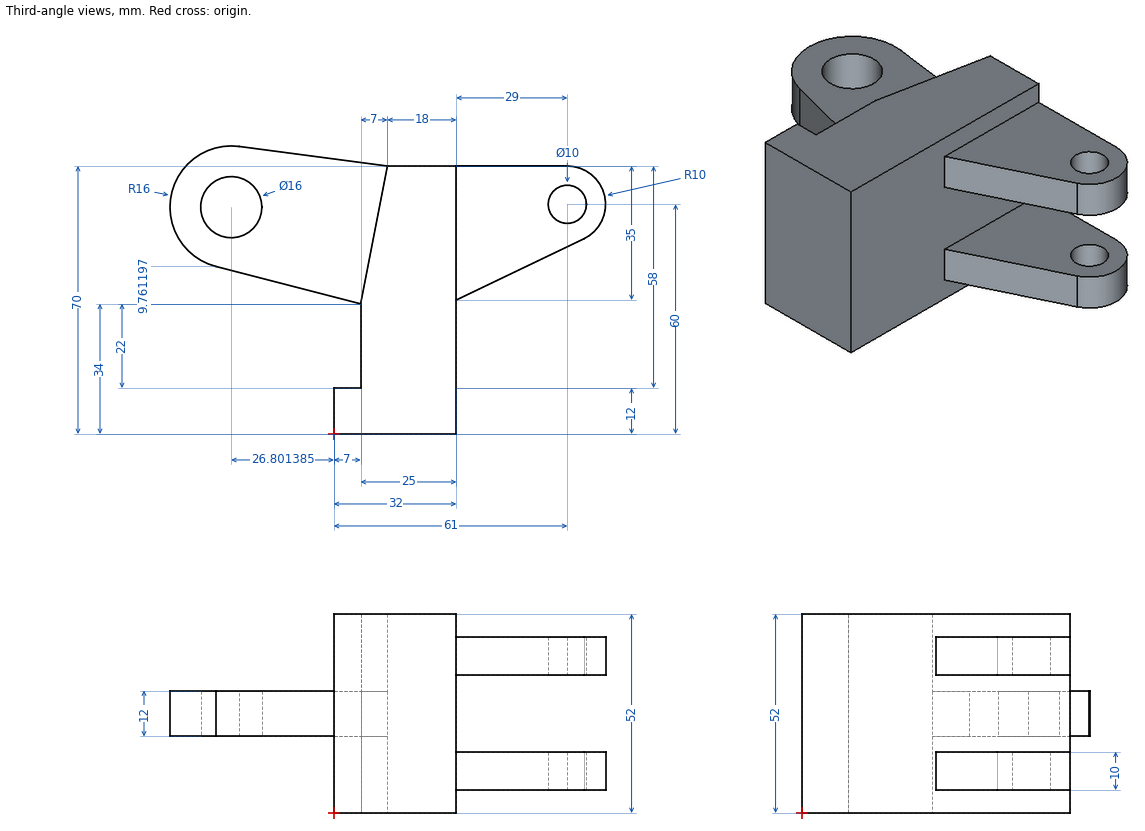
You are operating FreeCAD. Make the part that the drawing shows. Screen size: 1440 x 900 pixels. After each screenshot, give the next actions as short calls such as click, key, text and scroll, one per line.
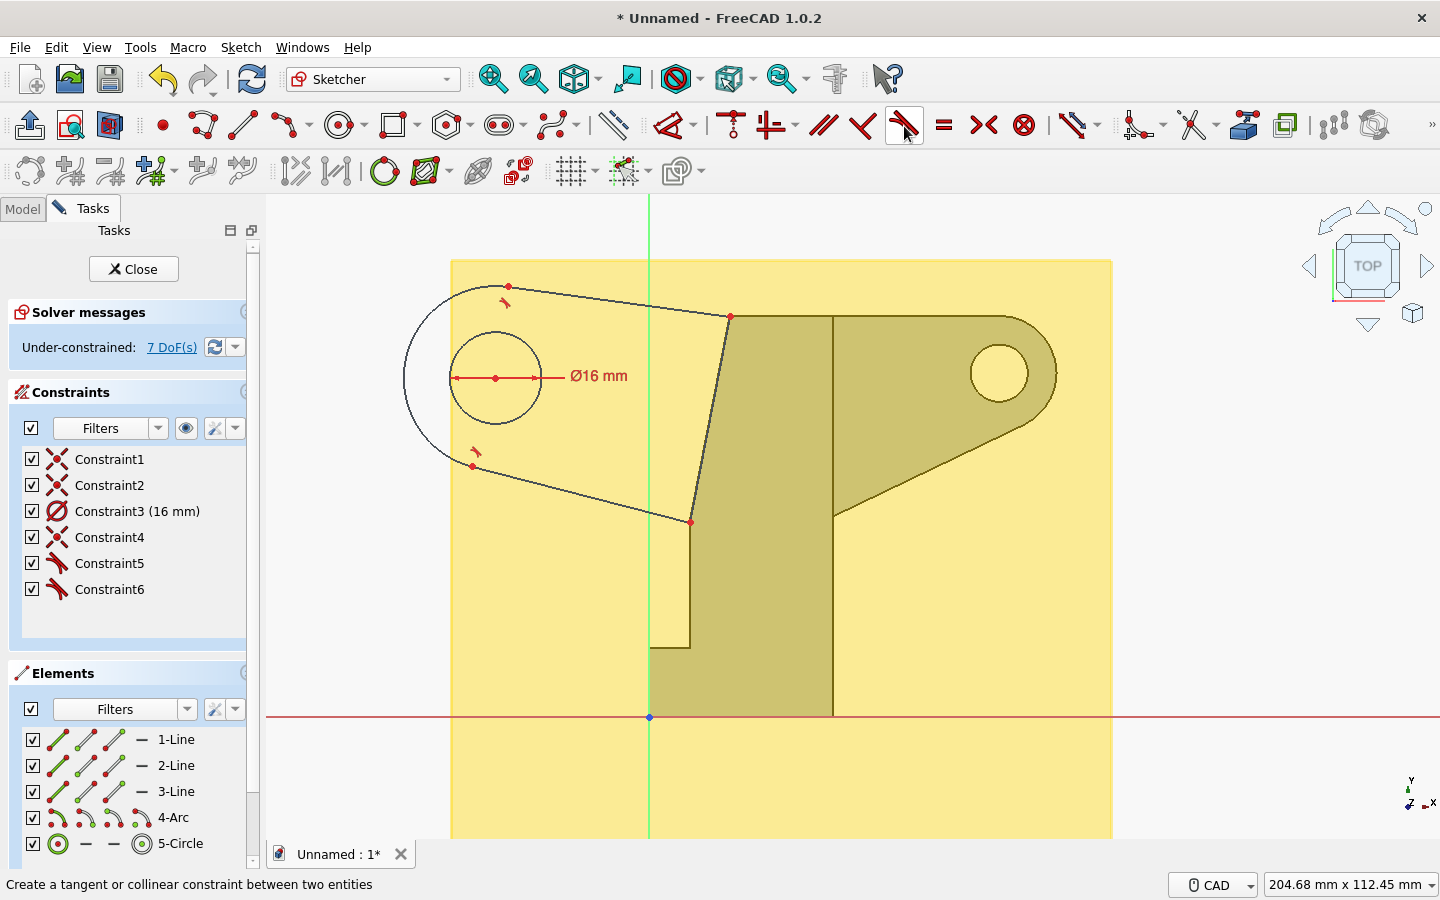
click(668, 126)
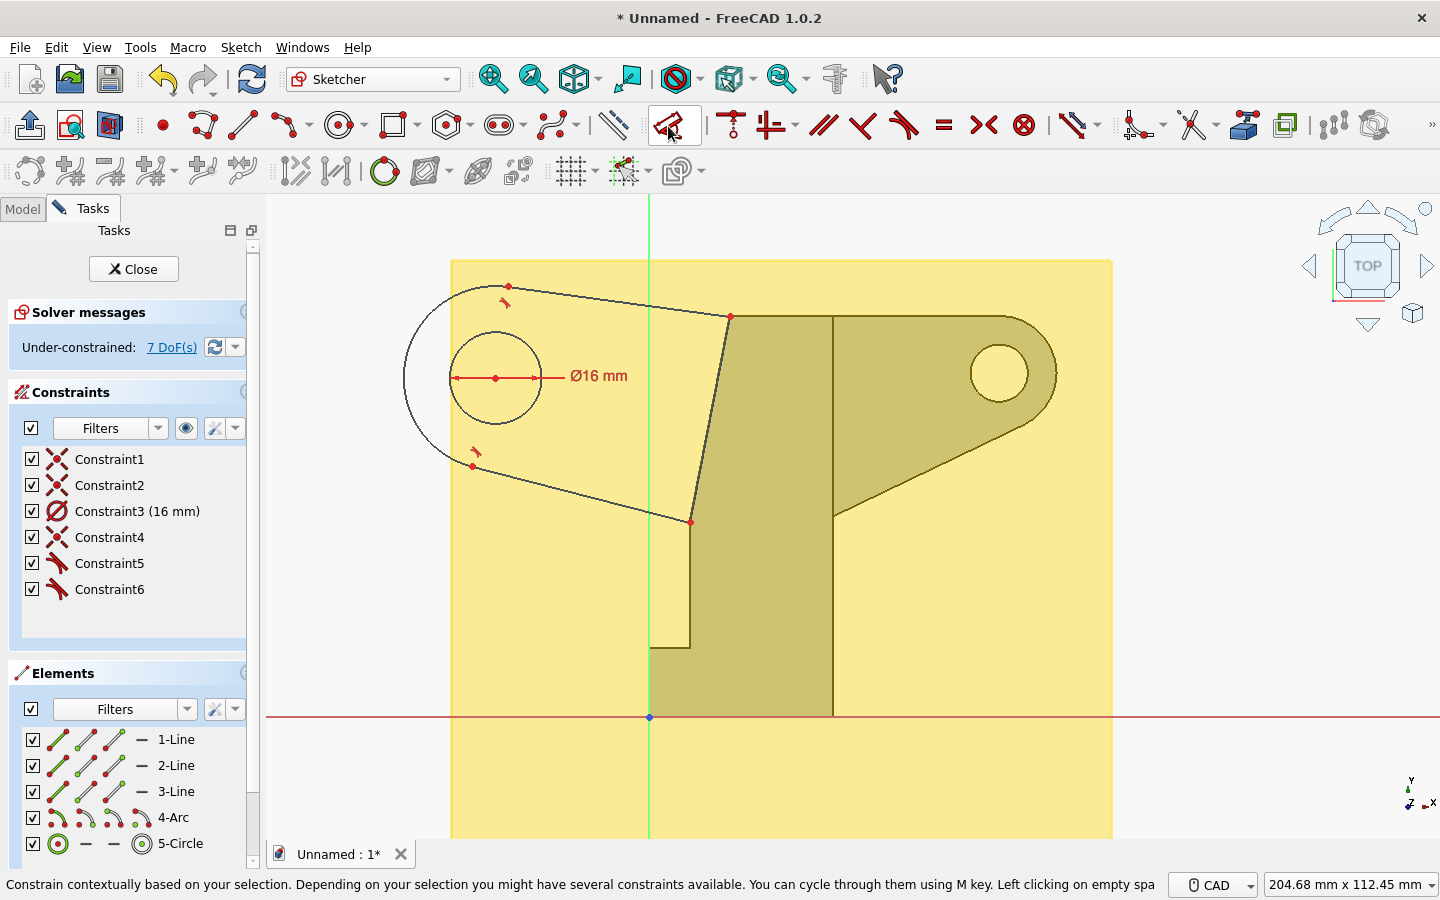
click(432, 312)
click(410, 289)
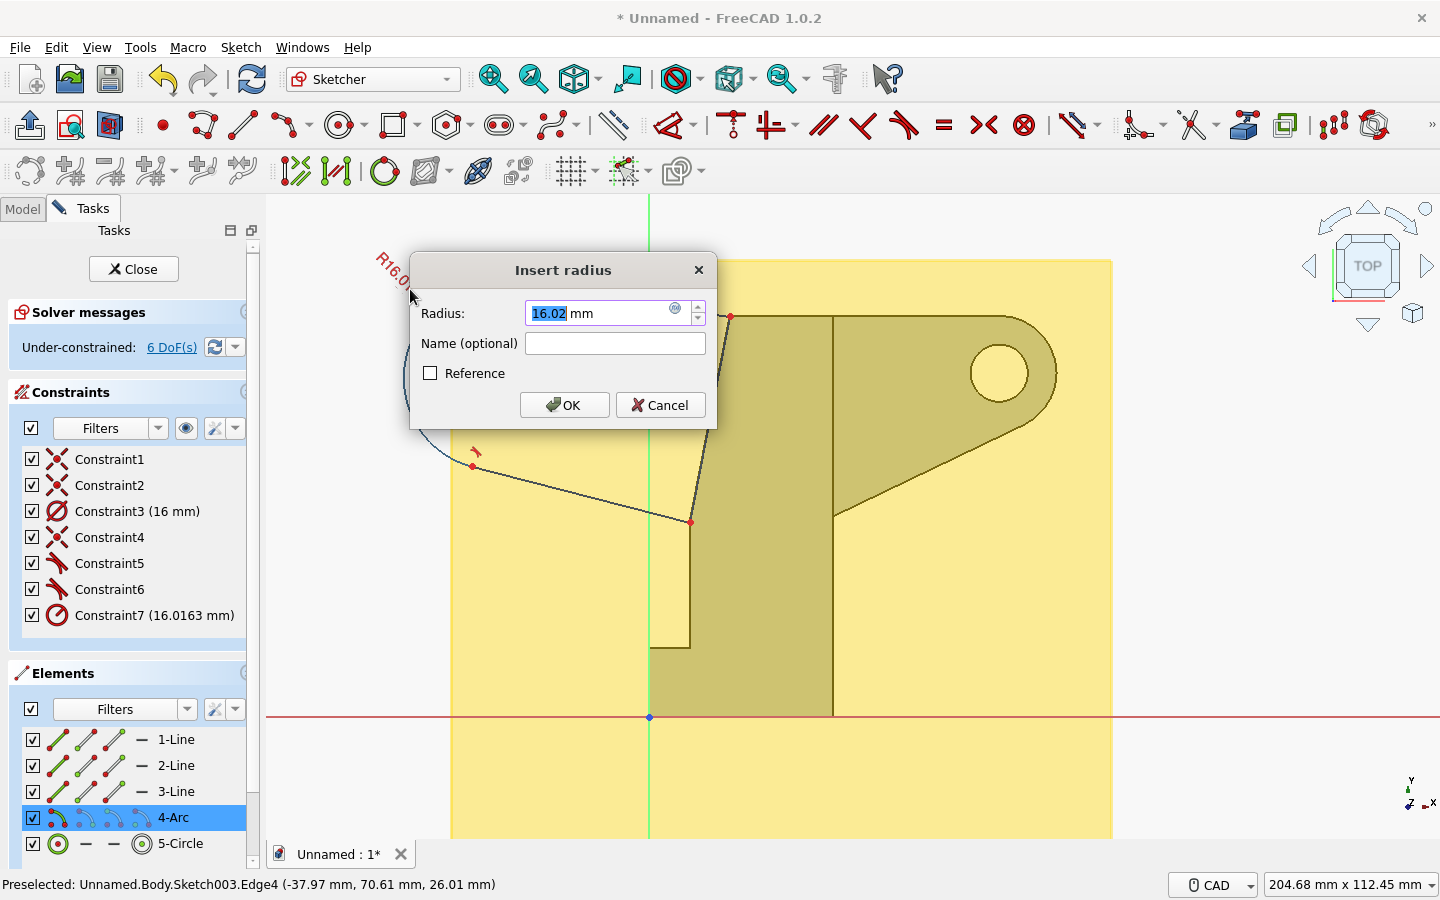
text(16)
key(Return)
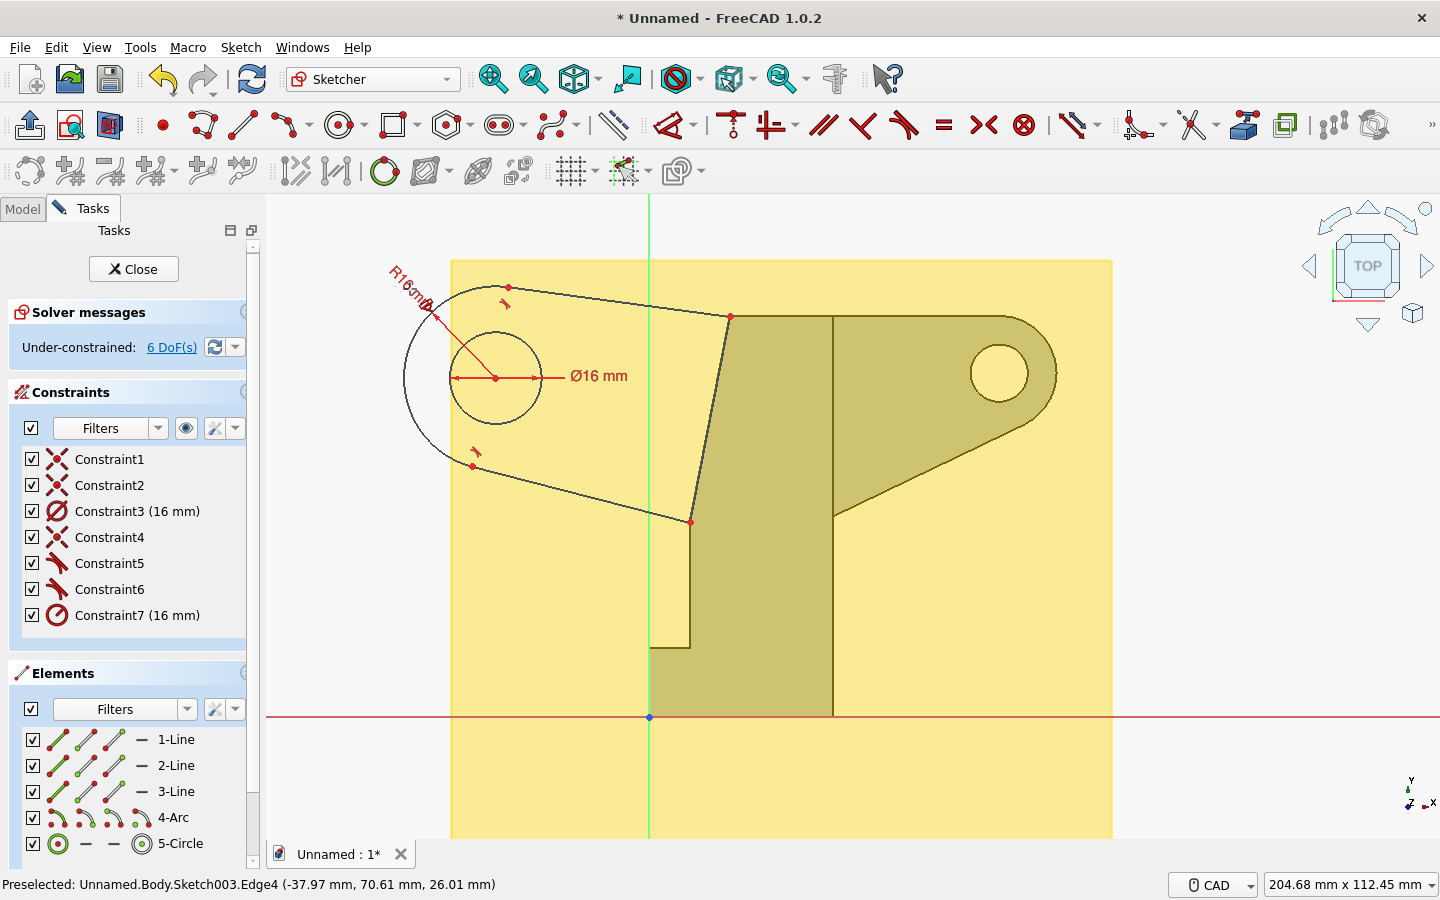
click(690, 523)
click(670, 751)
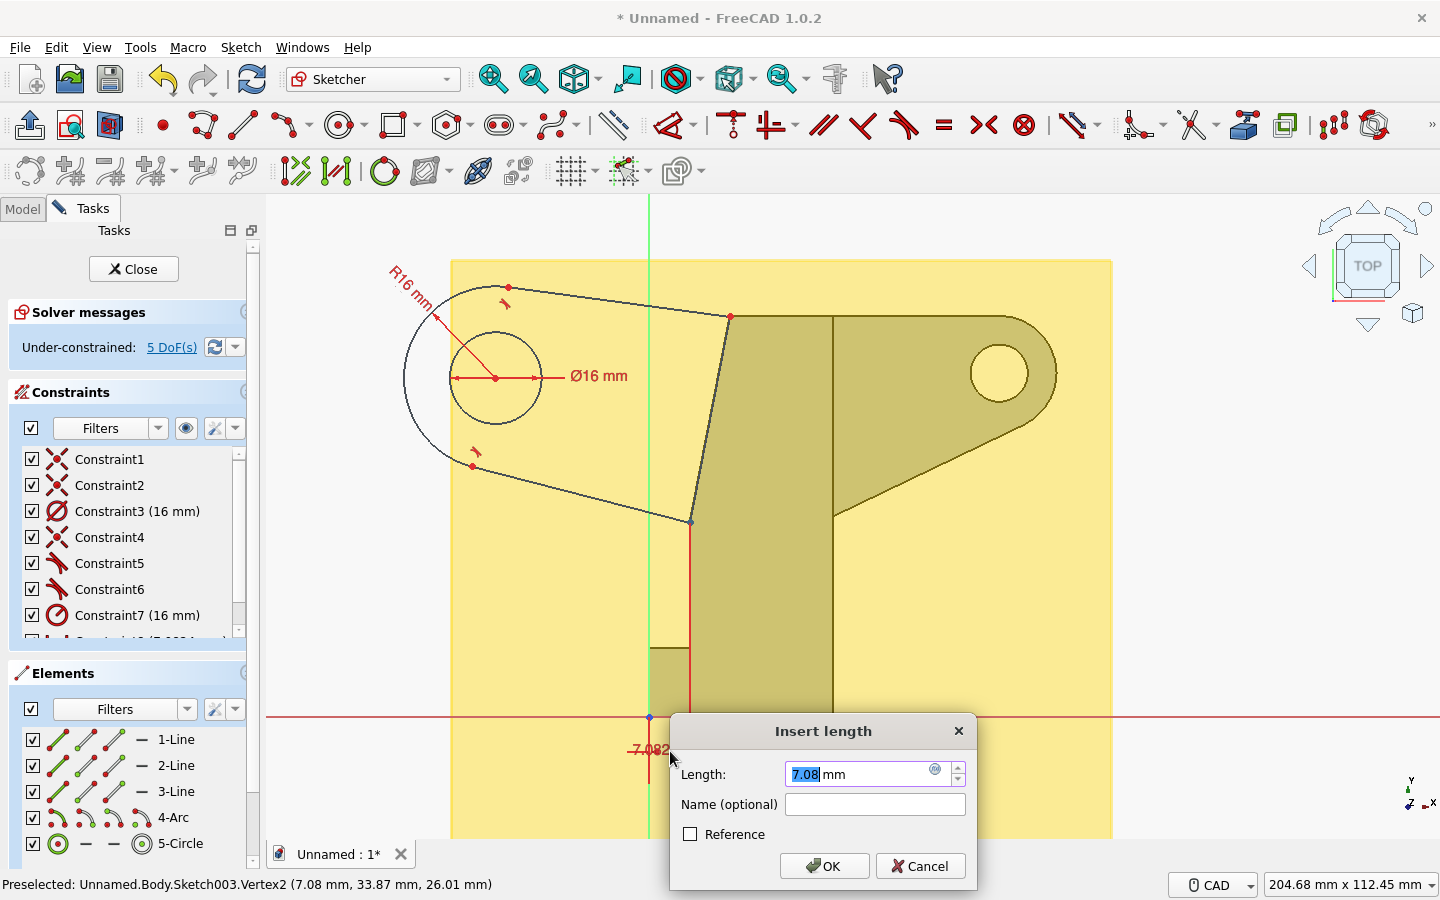
text(7)
key(Return)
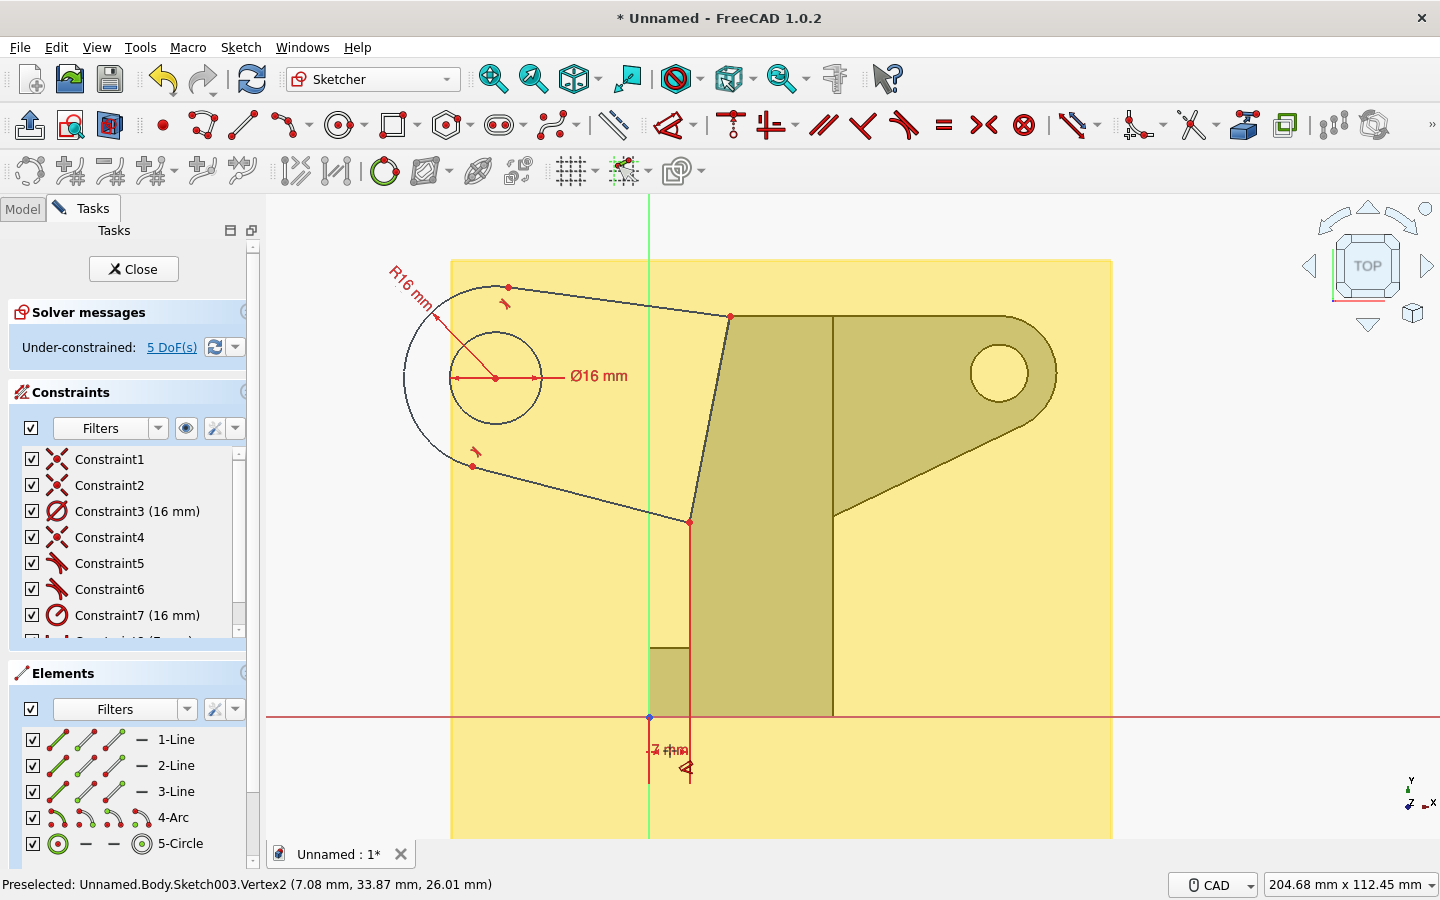
click(702, 461)
click(710, 283)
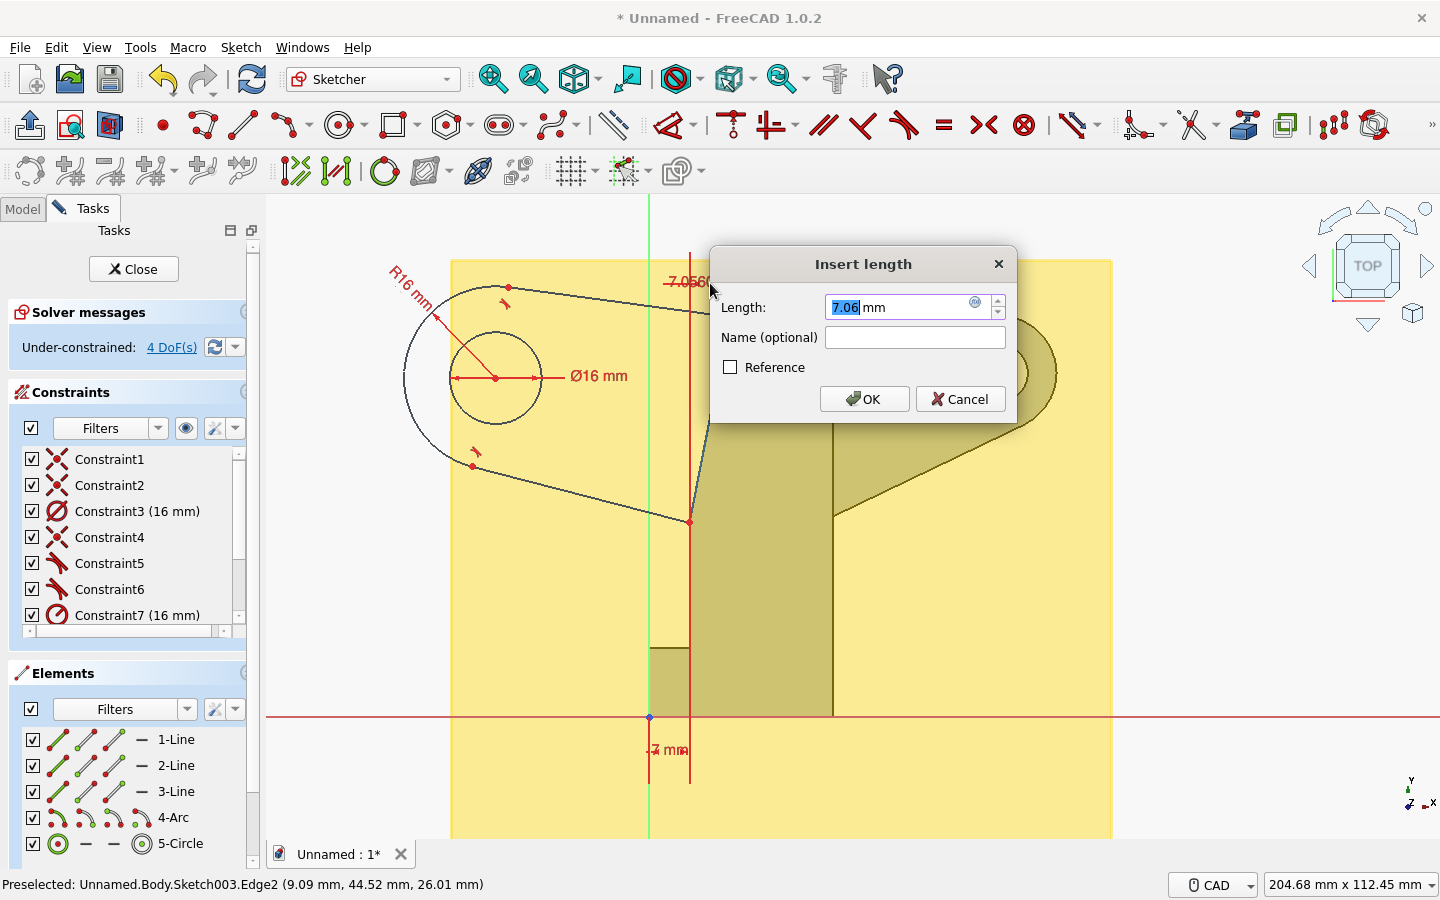
text(7)
key(Return)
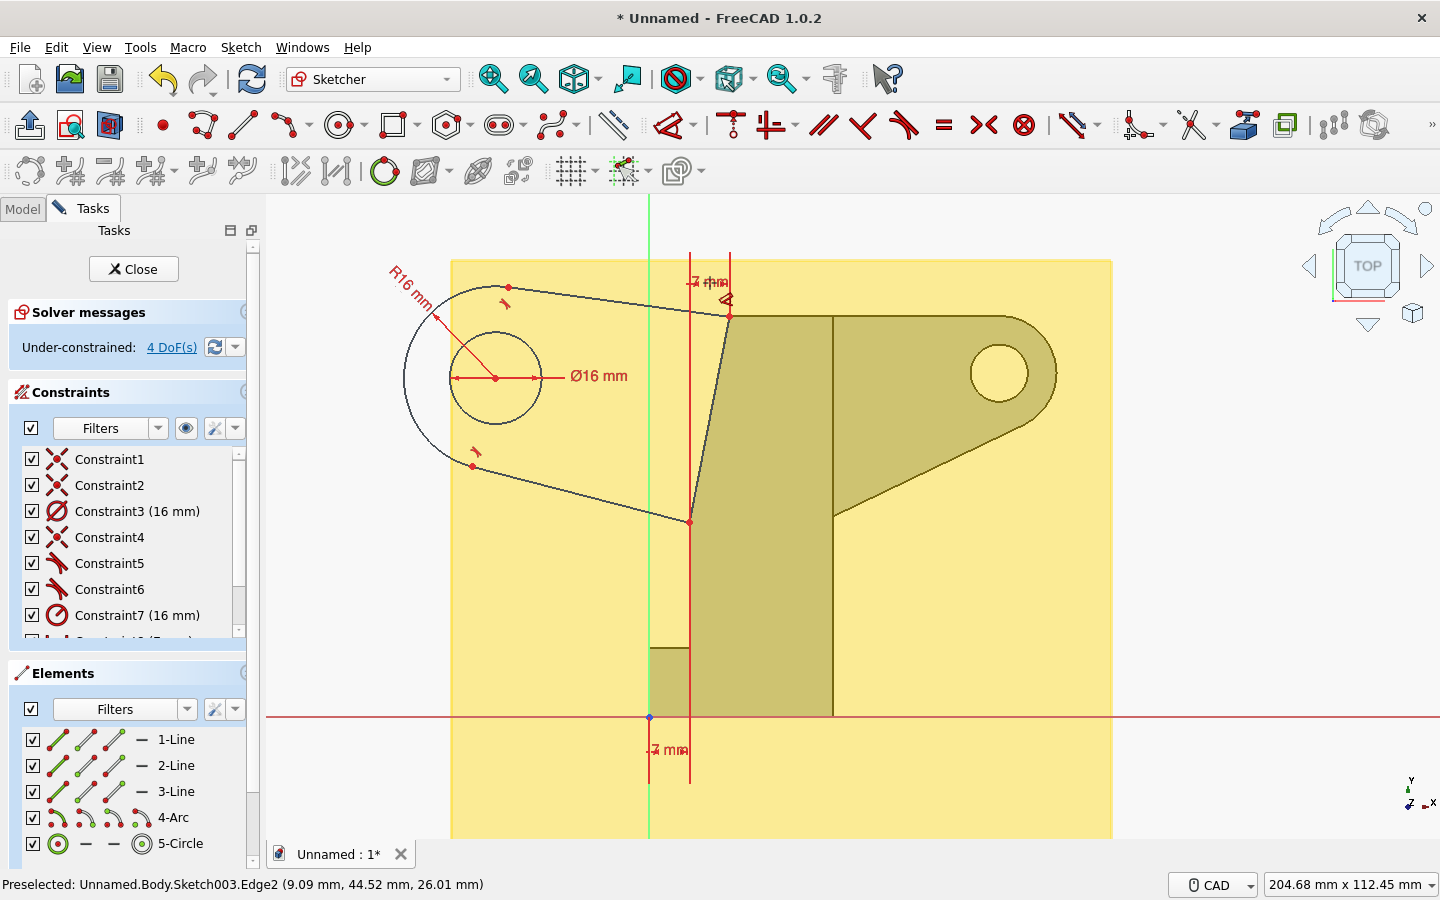
click(690, 523)
click(724, 620)